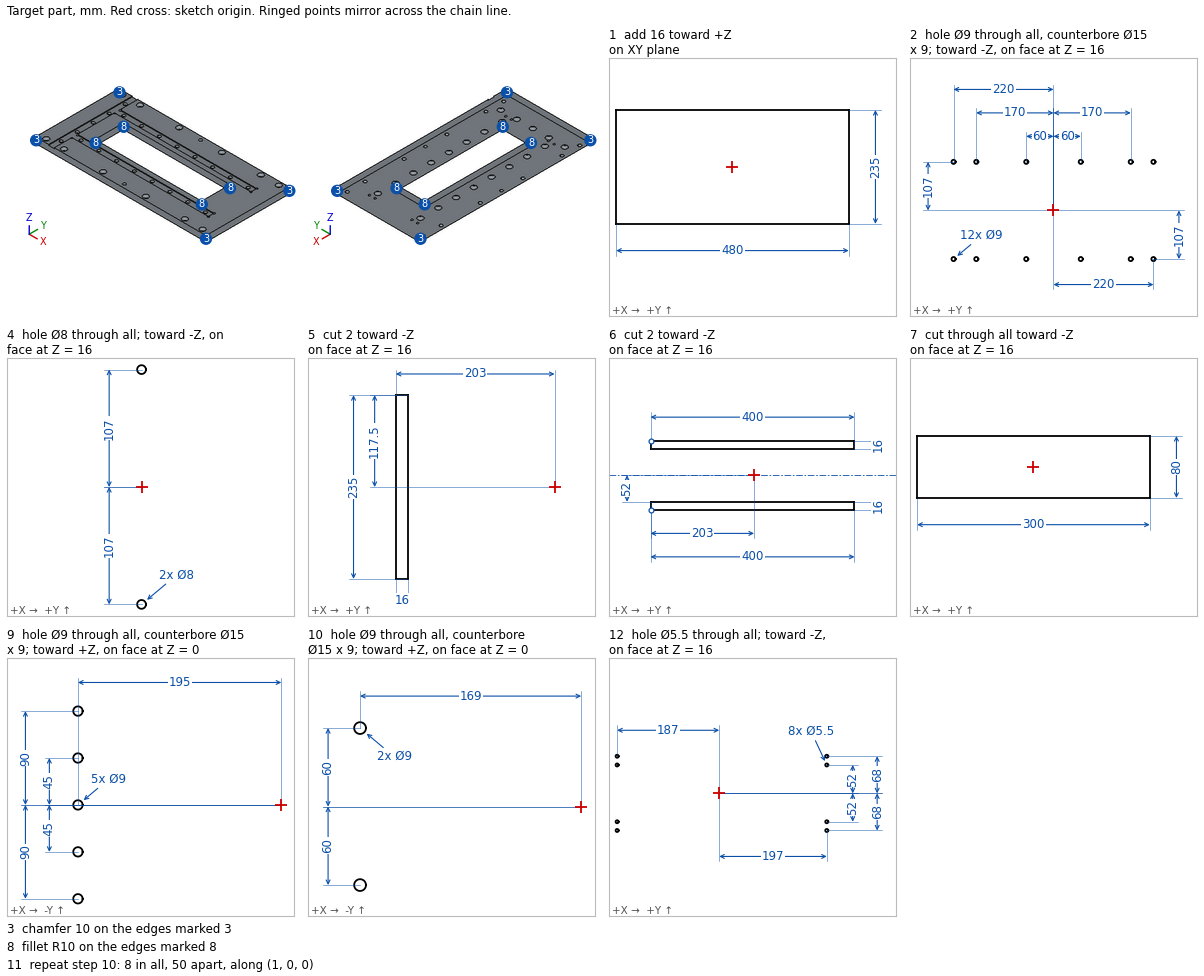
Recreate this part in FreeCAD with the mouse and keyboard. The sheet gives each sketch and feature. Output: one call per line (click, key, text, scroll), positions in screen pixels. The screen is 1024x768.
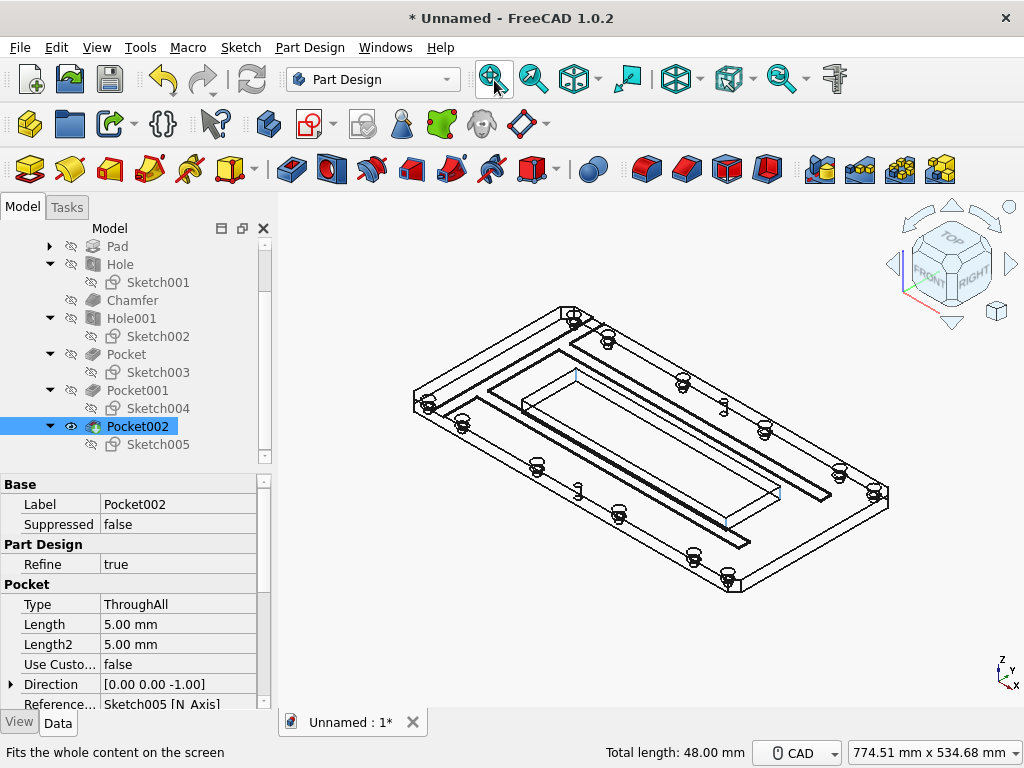
key(2)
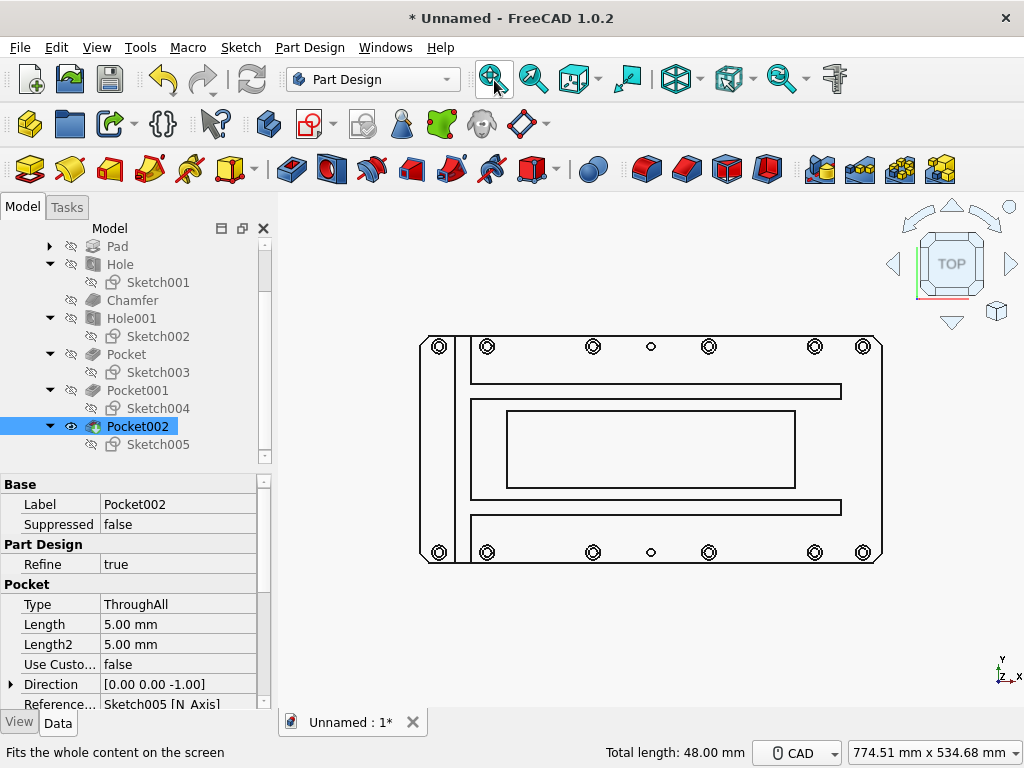
scroll(507, 487, up, 6)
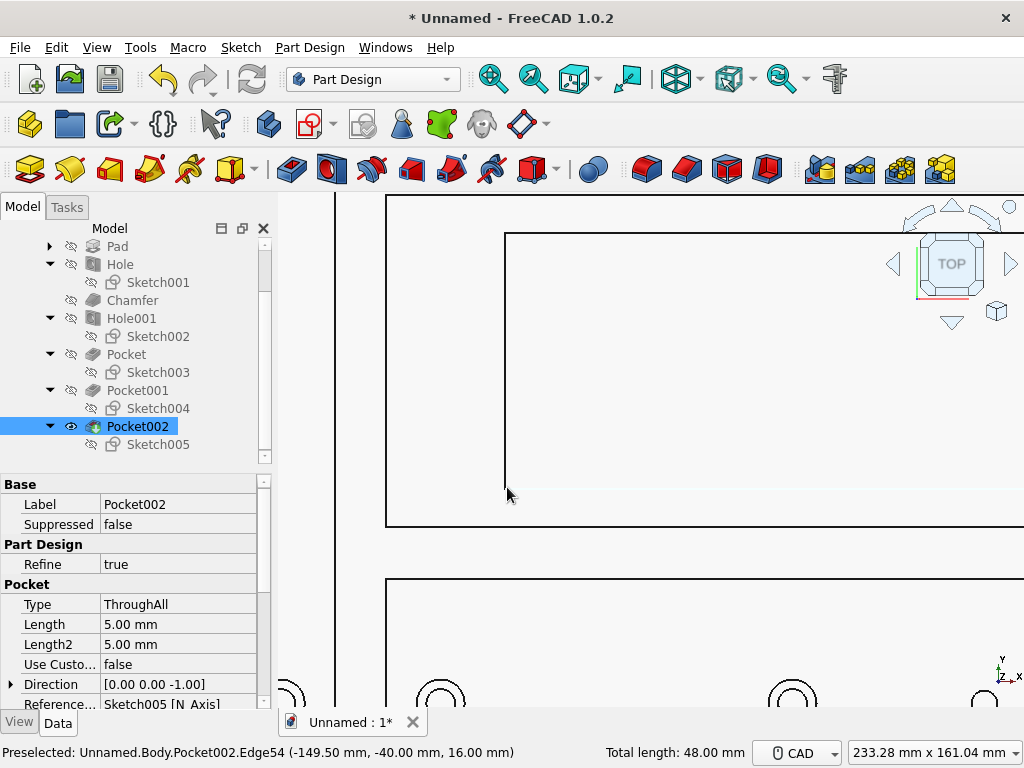
click(494, 80)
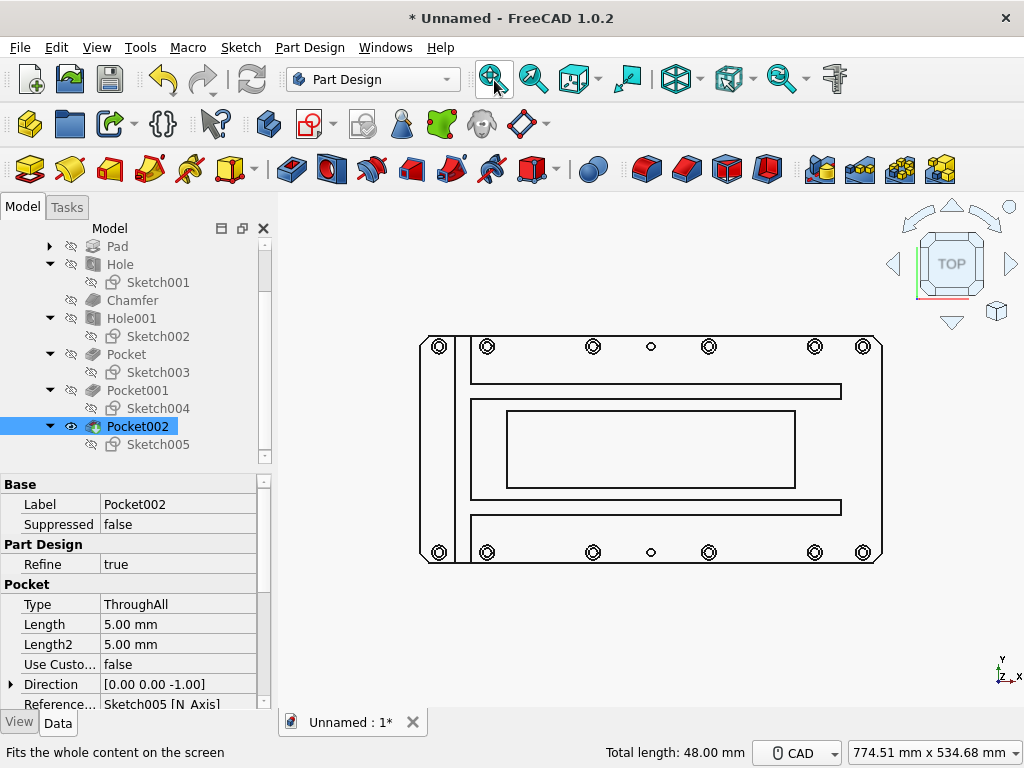
key(1)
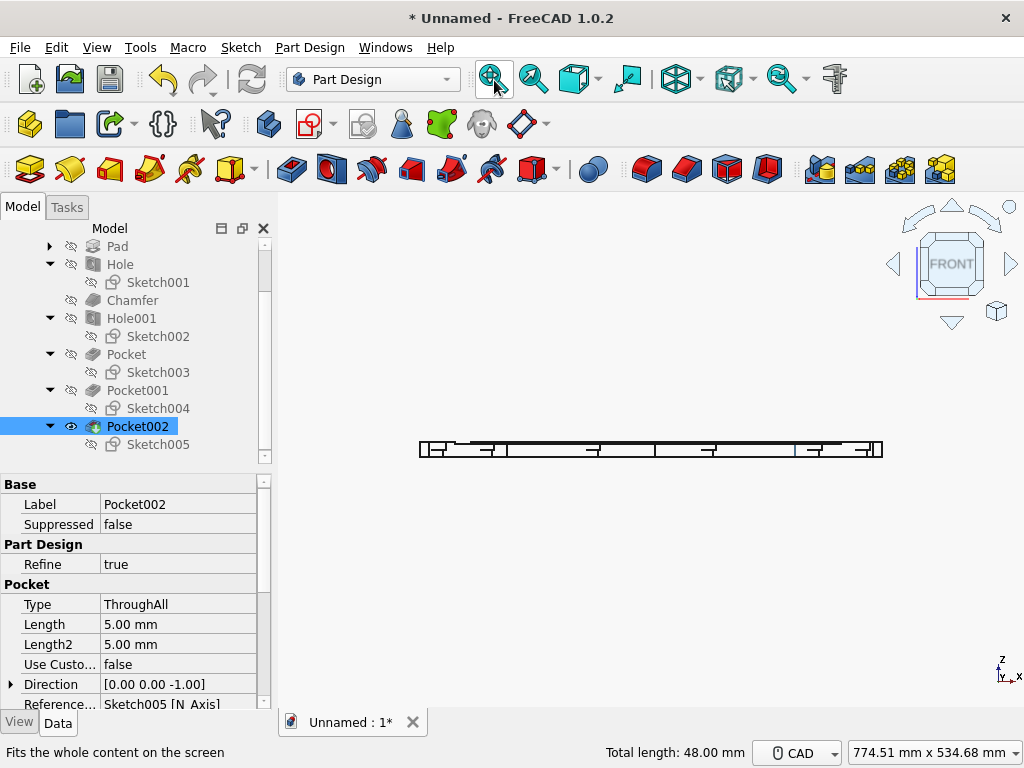
click(507, 449, ctrl)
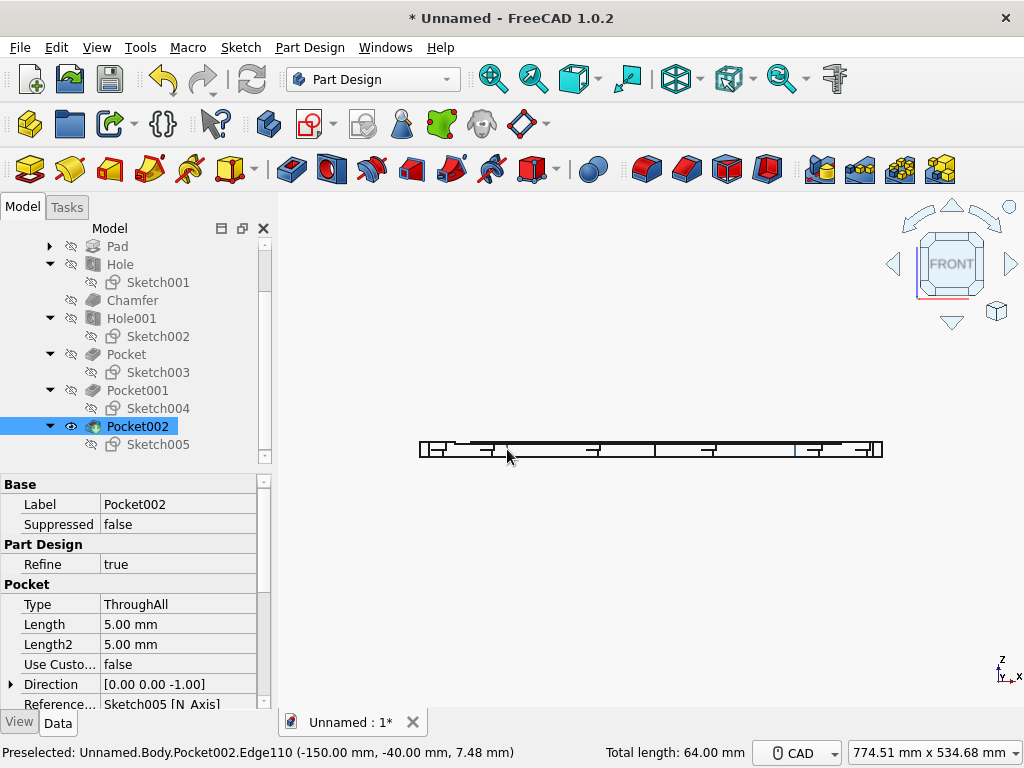
key(v)
key(1)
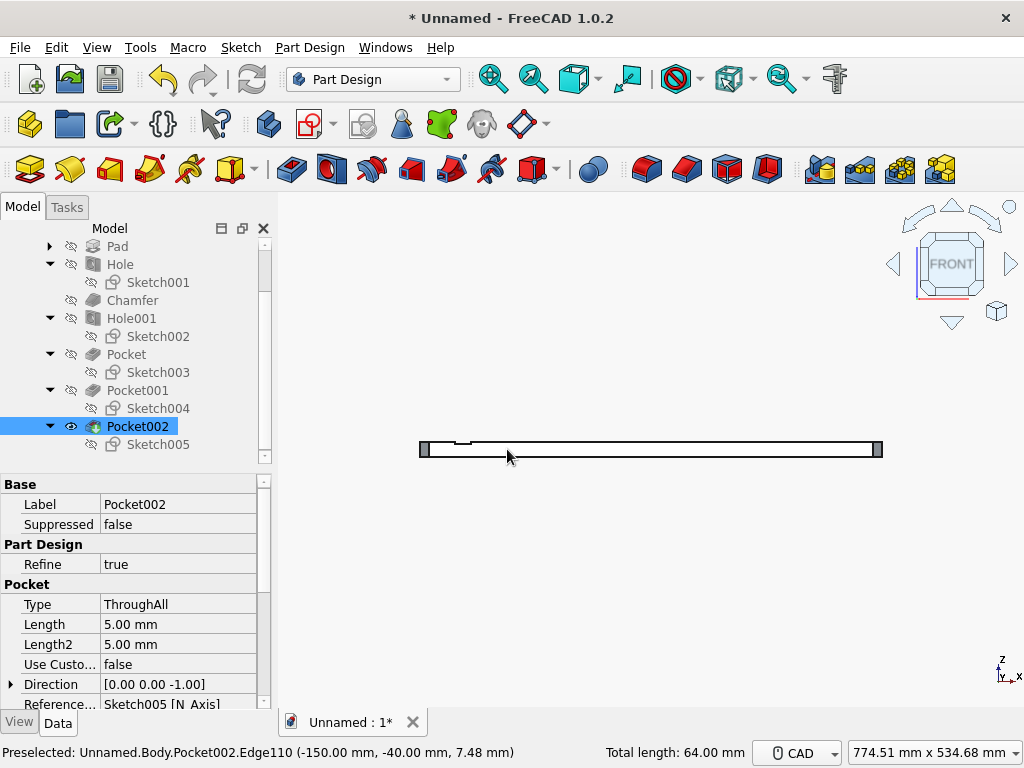
click(648, 170)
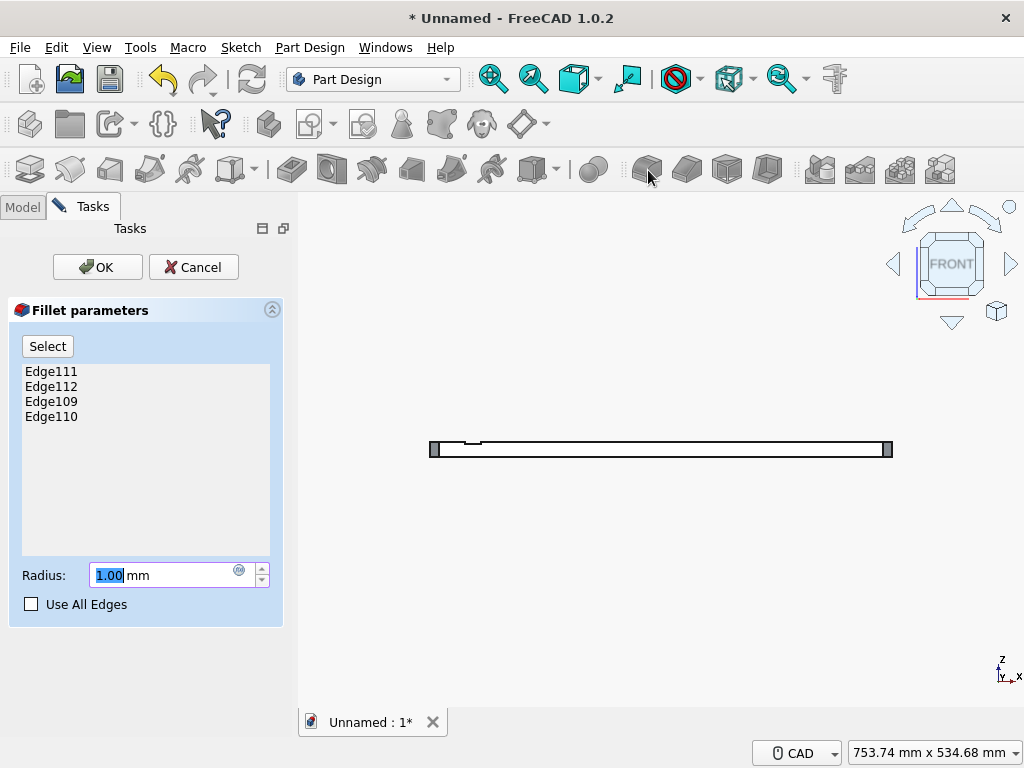
text(10)
key(Tab)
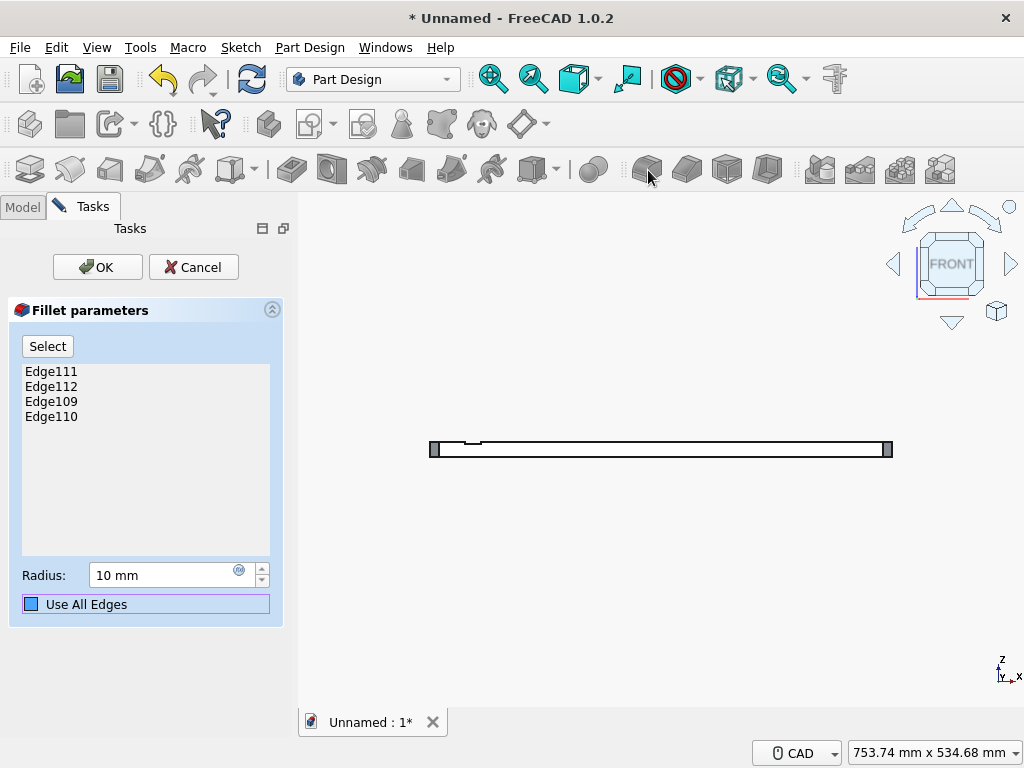
click(98, 267)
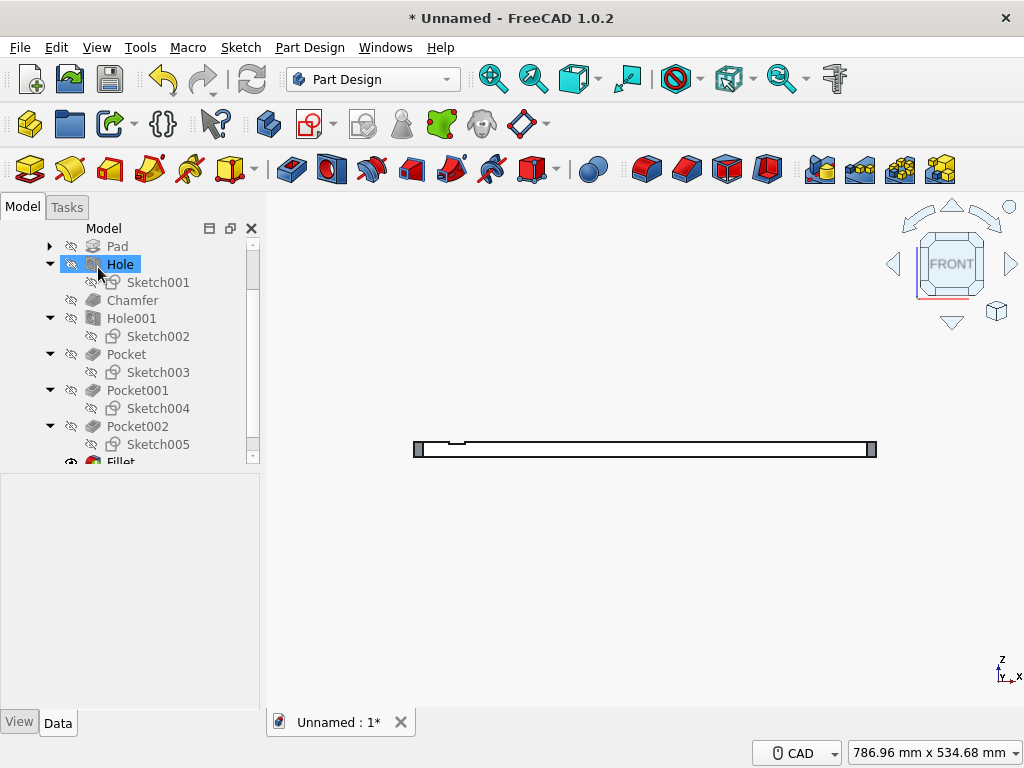
key(5)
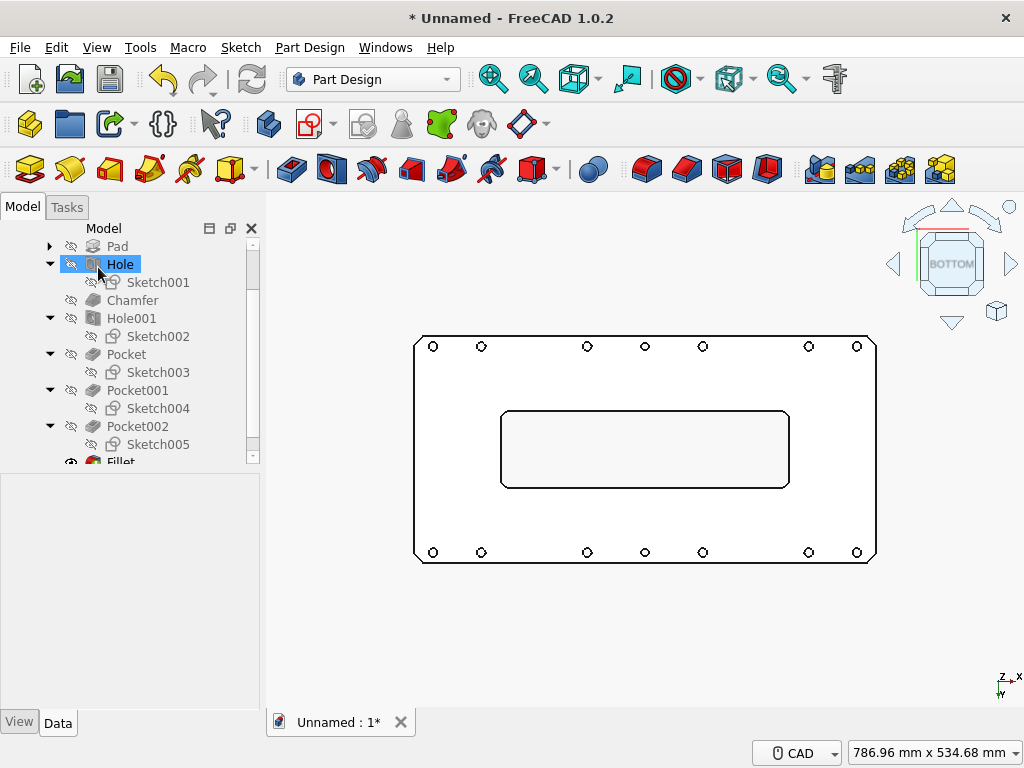
click(843, 513)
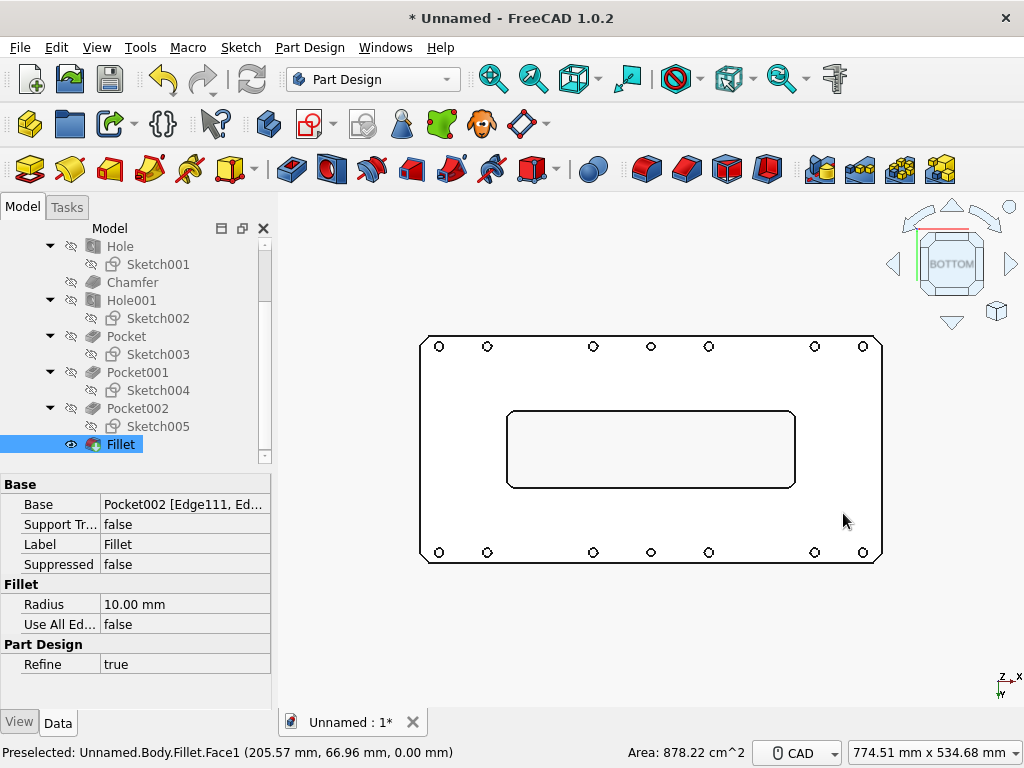
click(310, 124)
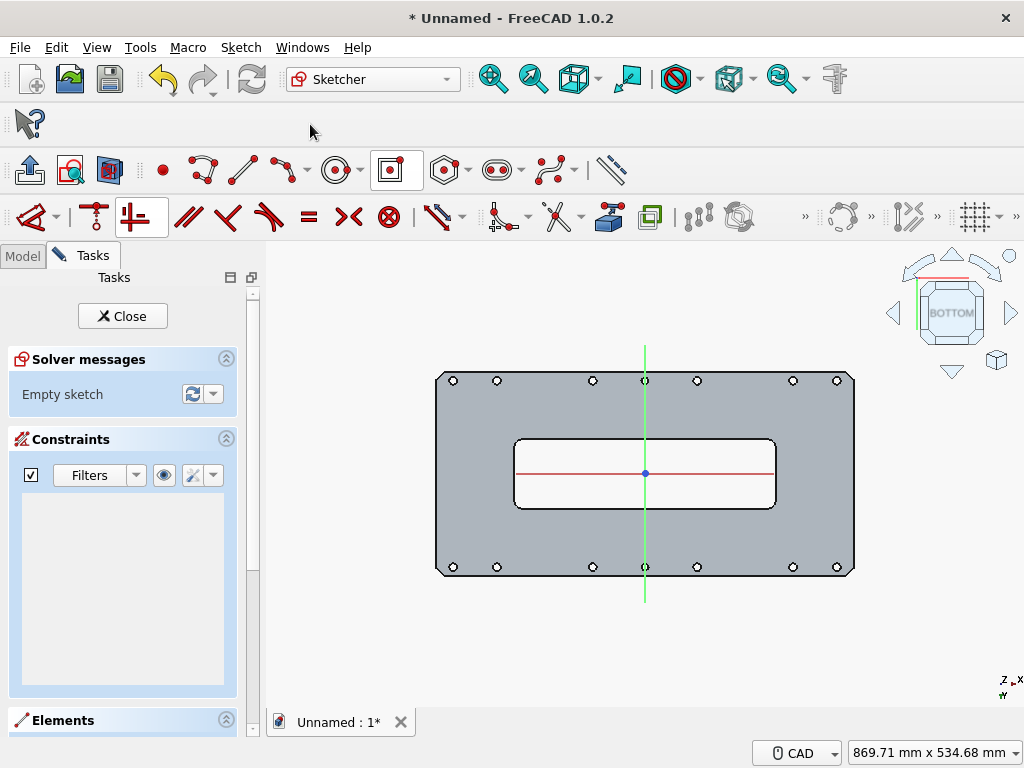
scroll(536, 474, up, 3)